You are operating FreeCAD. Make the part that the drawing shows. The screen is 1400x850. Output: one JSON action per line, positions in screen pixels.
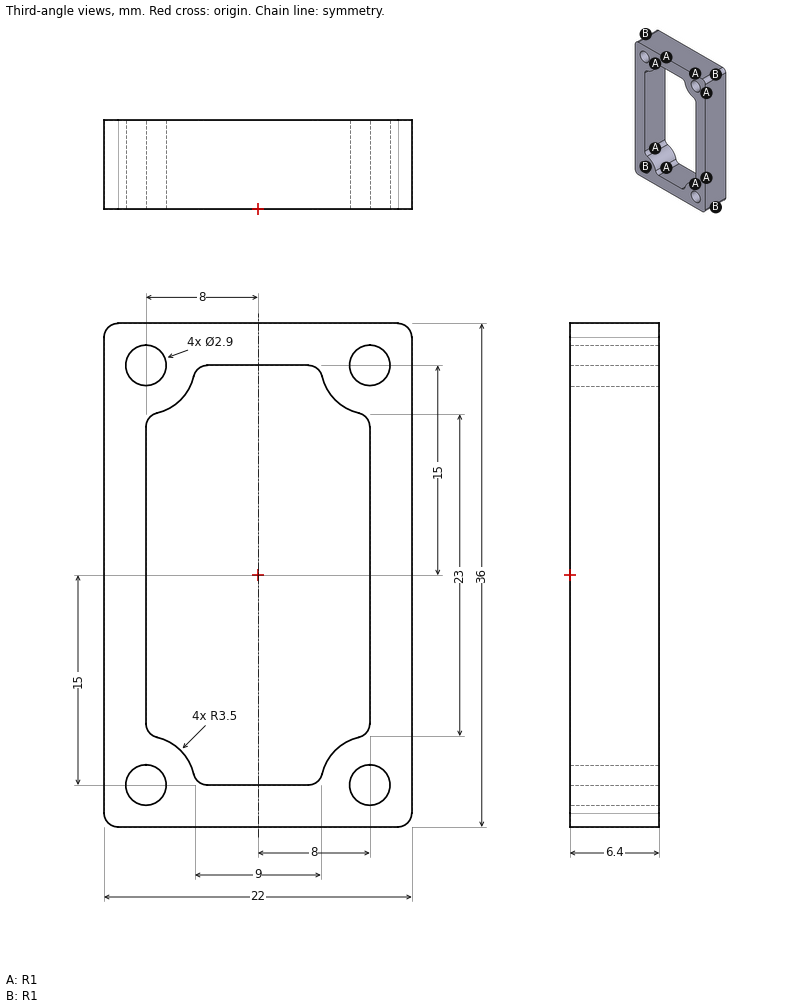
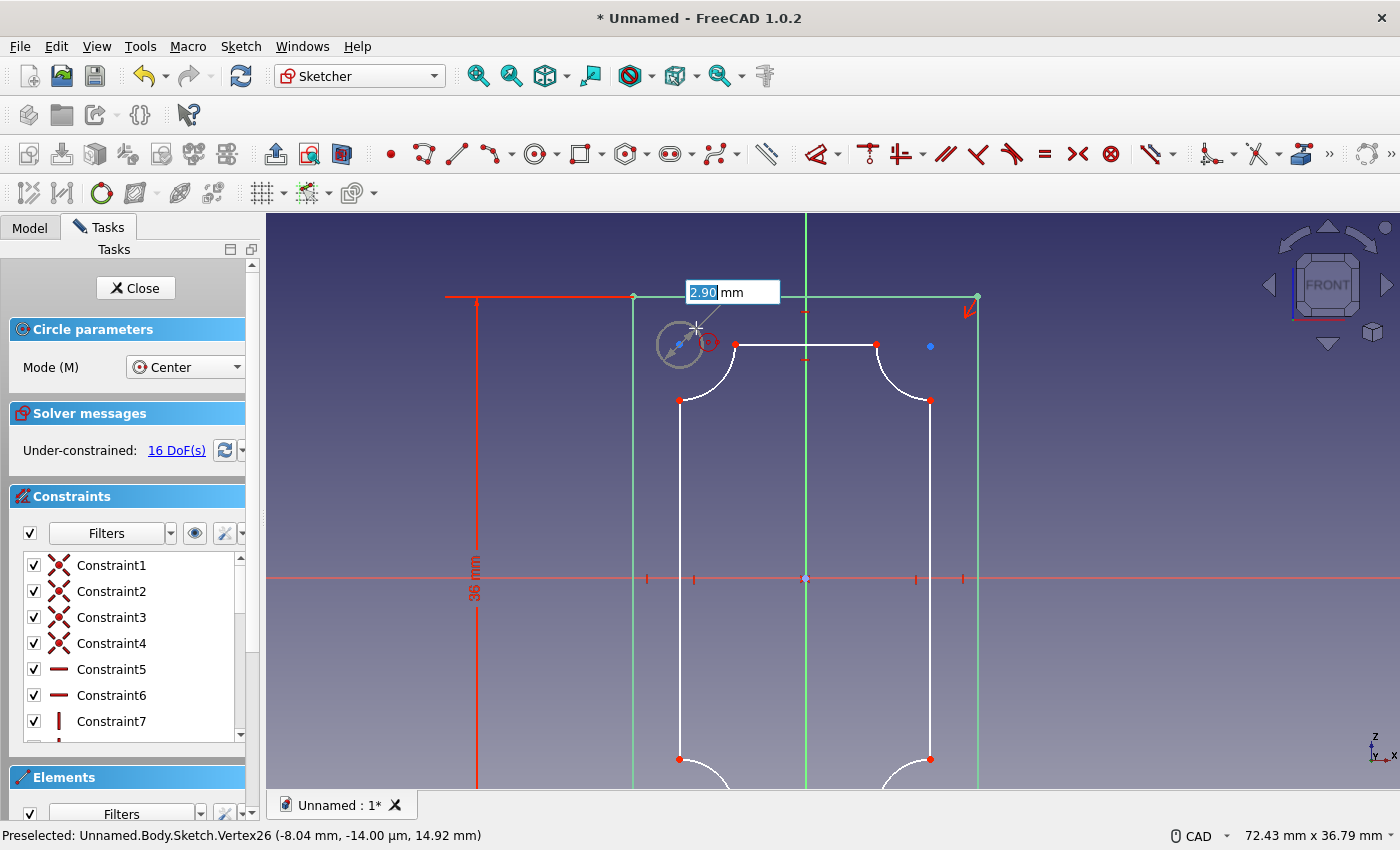
{"action": "type", "text": "2.9"}
{"action": "key", "text": "Return"}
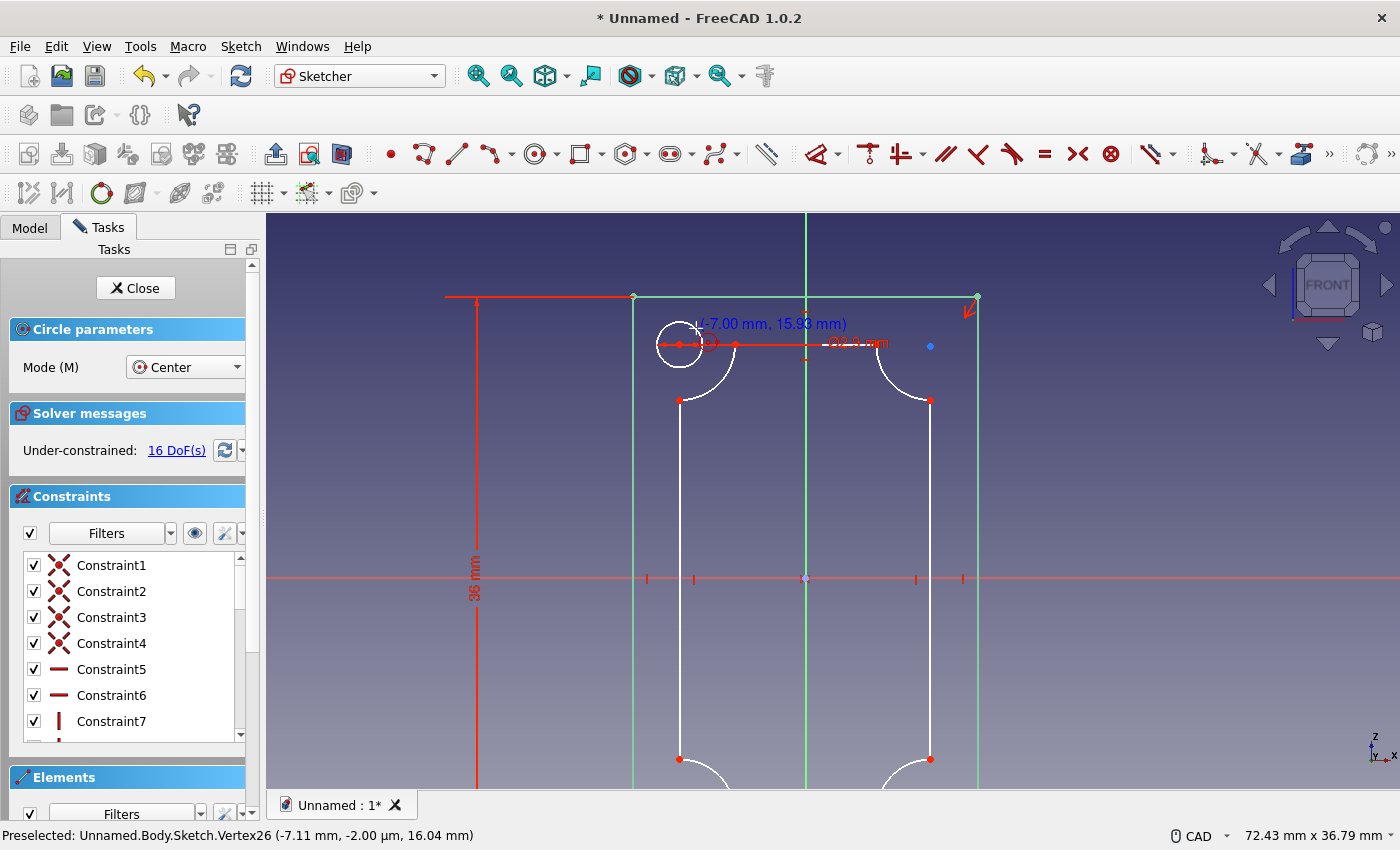
{"action": "left_click", "coordinate": [931, 344]}
{"action": "mouse_move", "coordinate": [947, 328]}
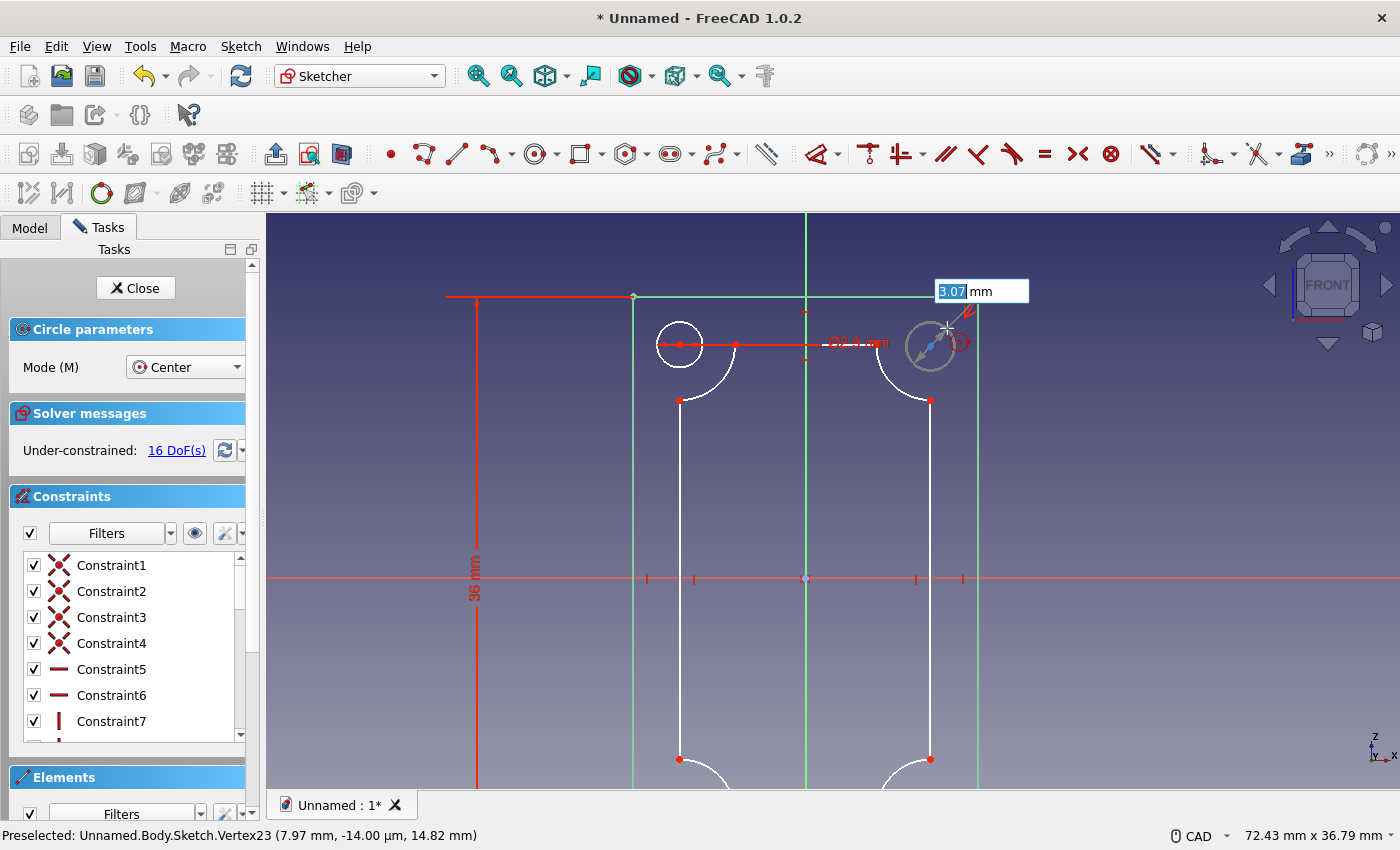
{"action": "type", "text": "2.9"}
{"action": "key", "text": "Return"}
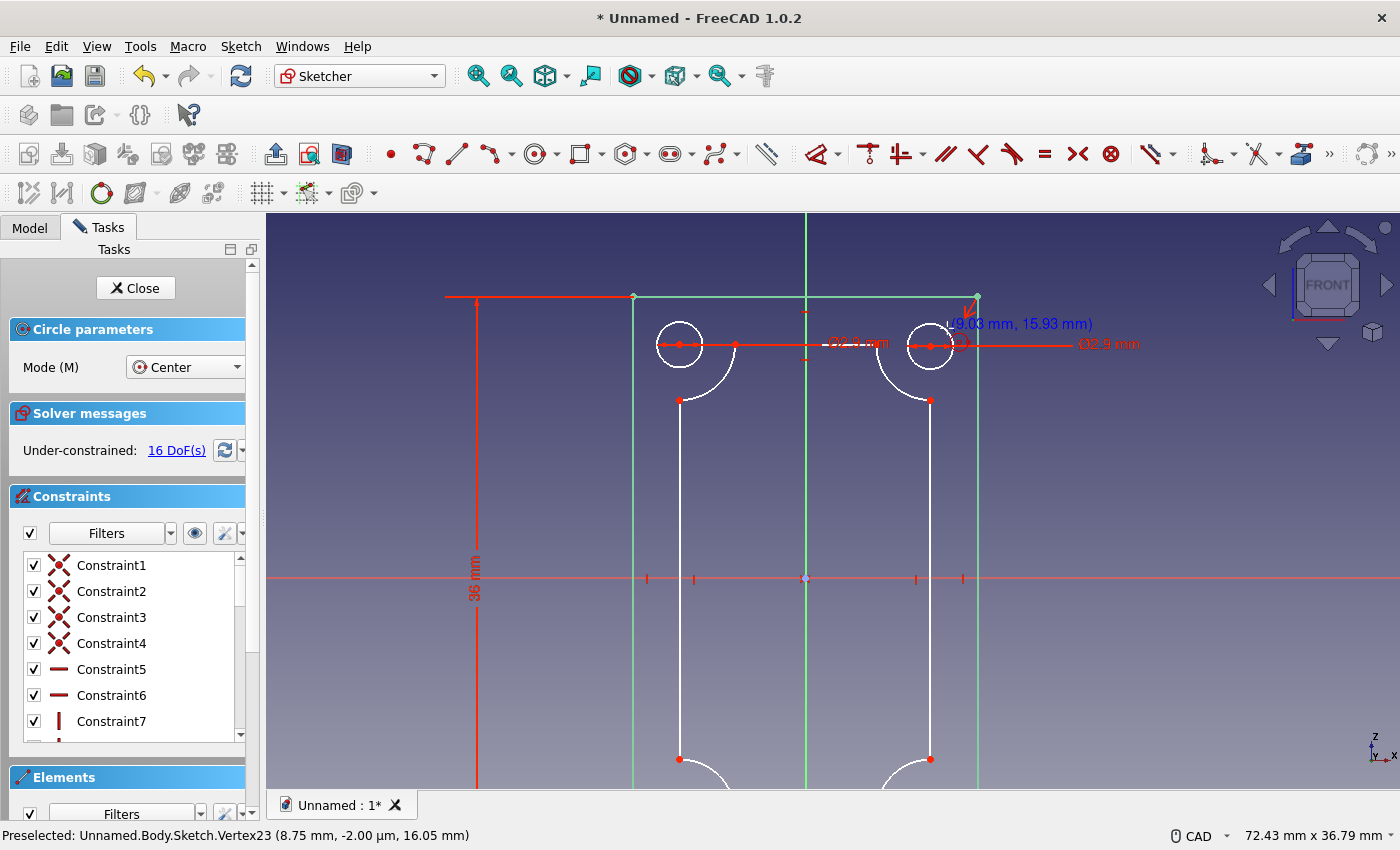
{"action": "scroll", "coordinate": [681, 343], "scroll_direction": "down", "scroll_amount": 2}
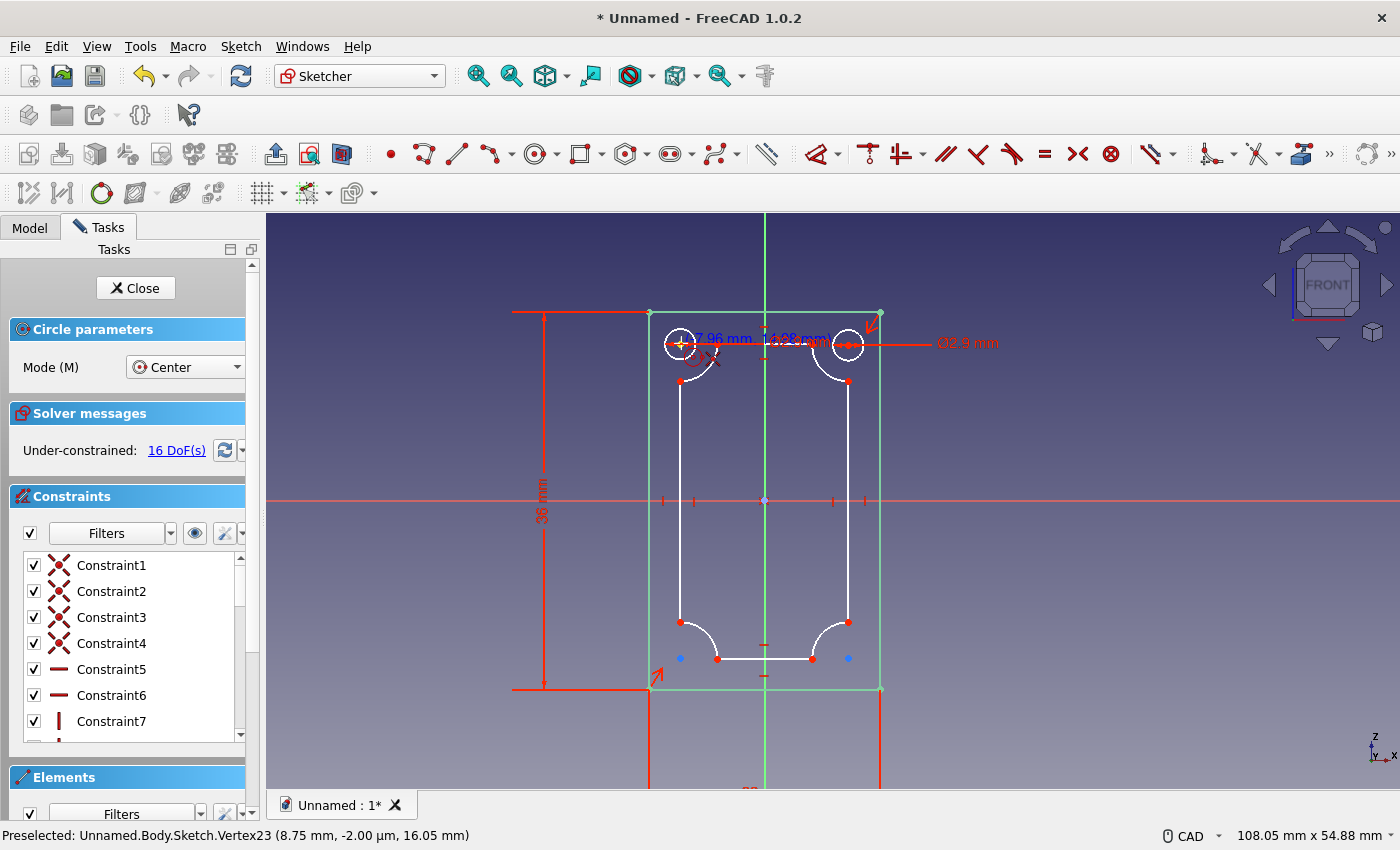
{"action": "scroll", "coordinate": [681, 658], "scroll_direction": "up", "scroll_amount": 2}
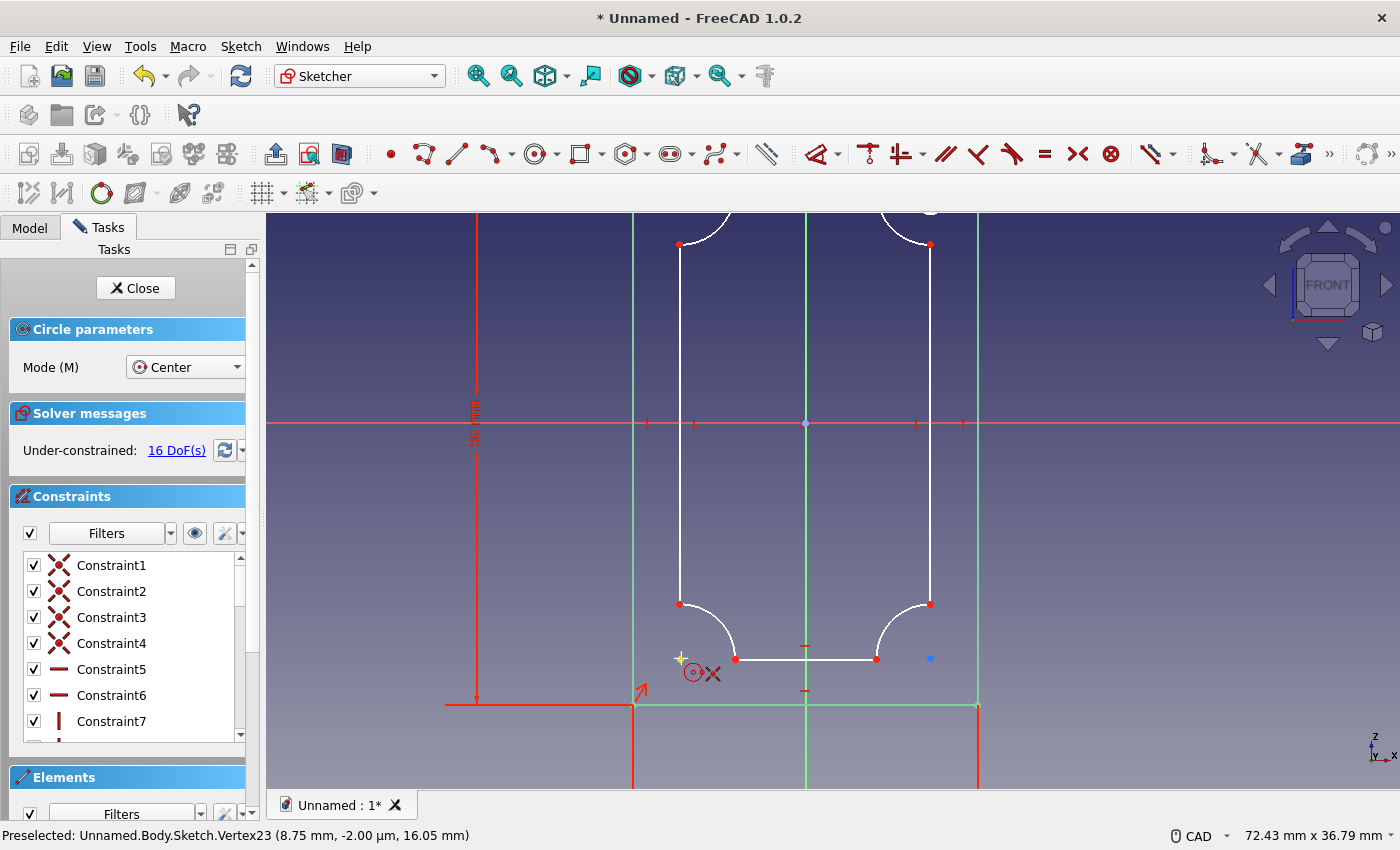
{"action": "left_click", "coordinate": [680, 658]}
{"action": "mouse_move", "coordinate": [696, 642]}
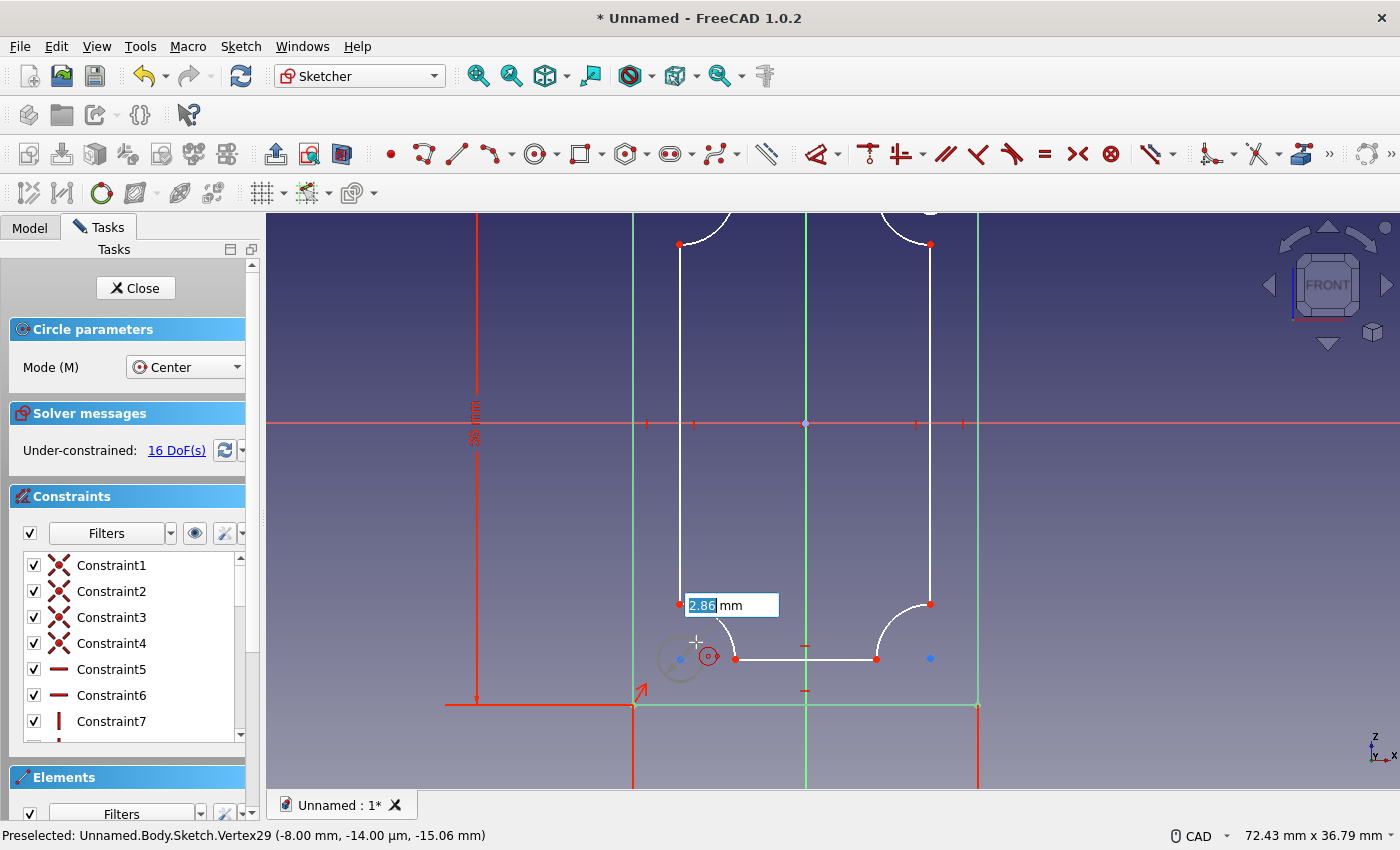
{"action": "type", "text": "2.9"}
{"action": "key", "text": "Return"}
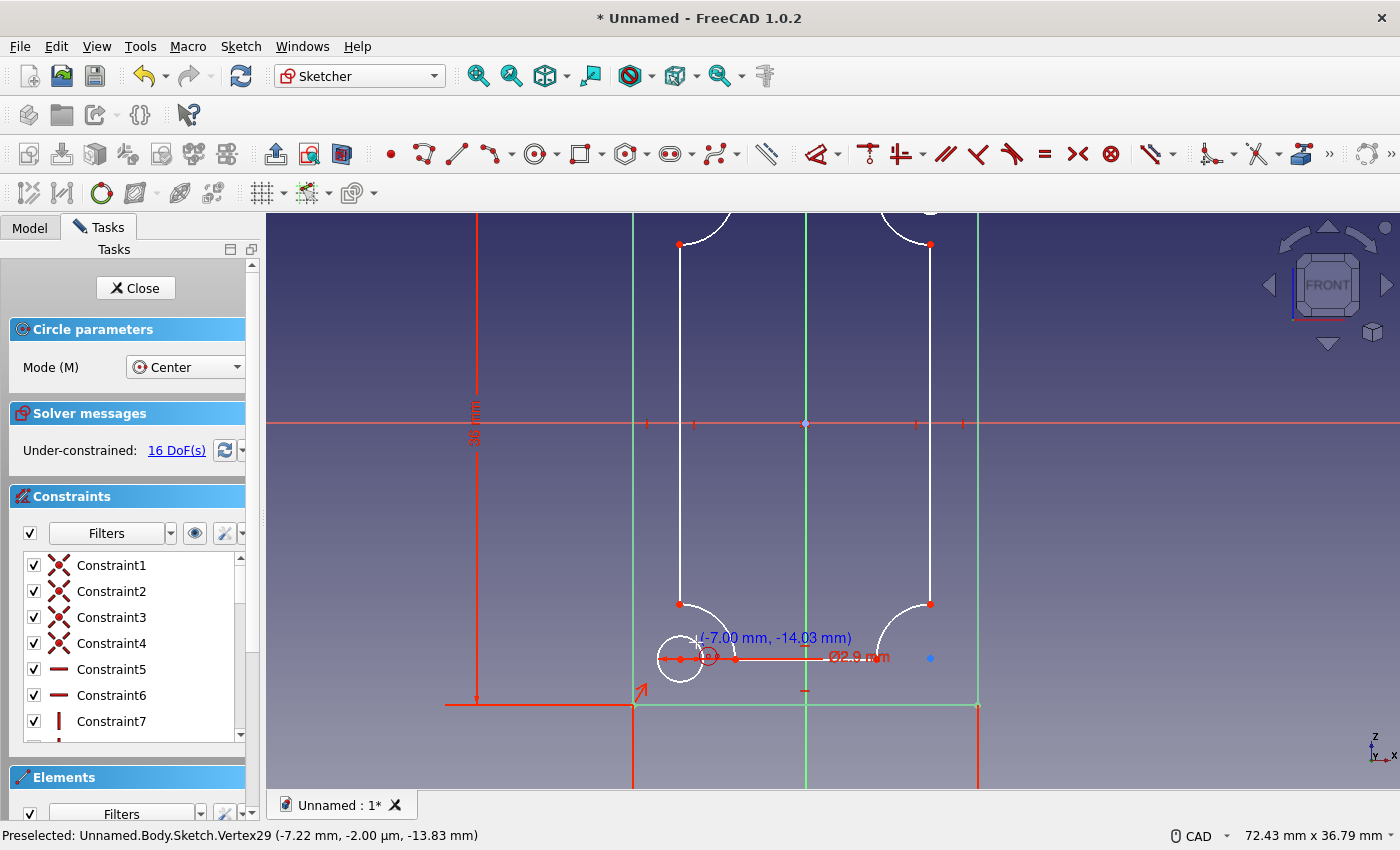
{"action": "left_click", "coordinate": [931, 658]}
{"action": "mouse_move", "coordinate": [947, 642]}